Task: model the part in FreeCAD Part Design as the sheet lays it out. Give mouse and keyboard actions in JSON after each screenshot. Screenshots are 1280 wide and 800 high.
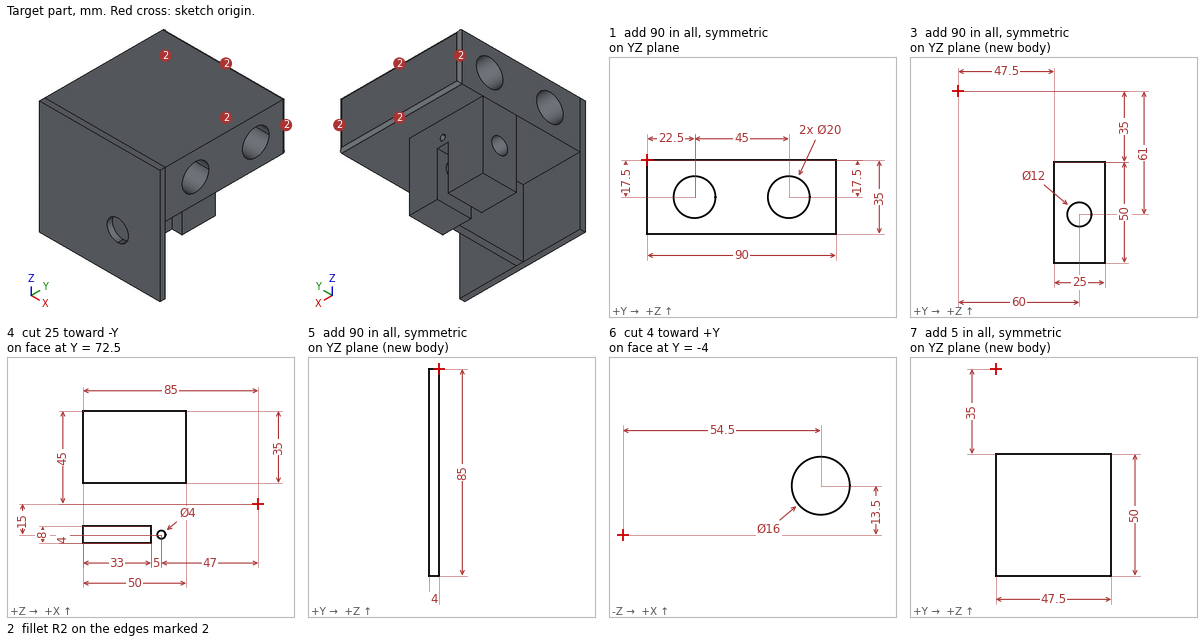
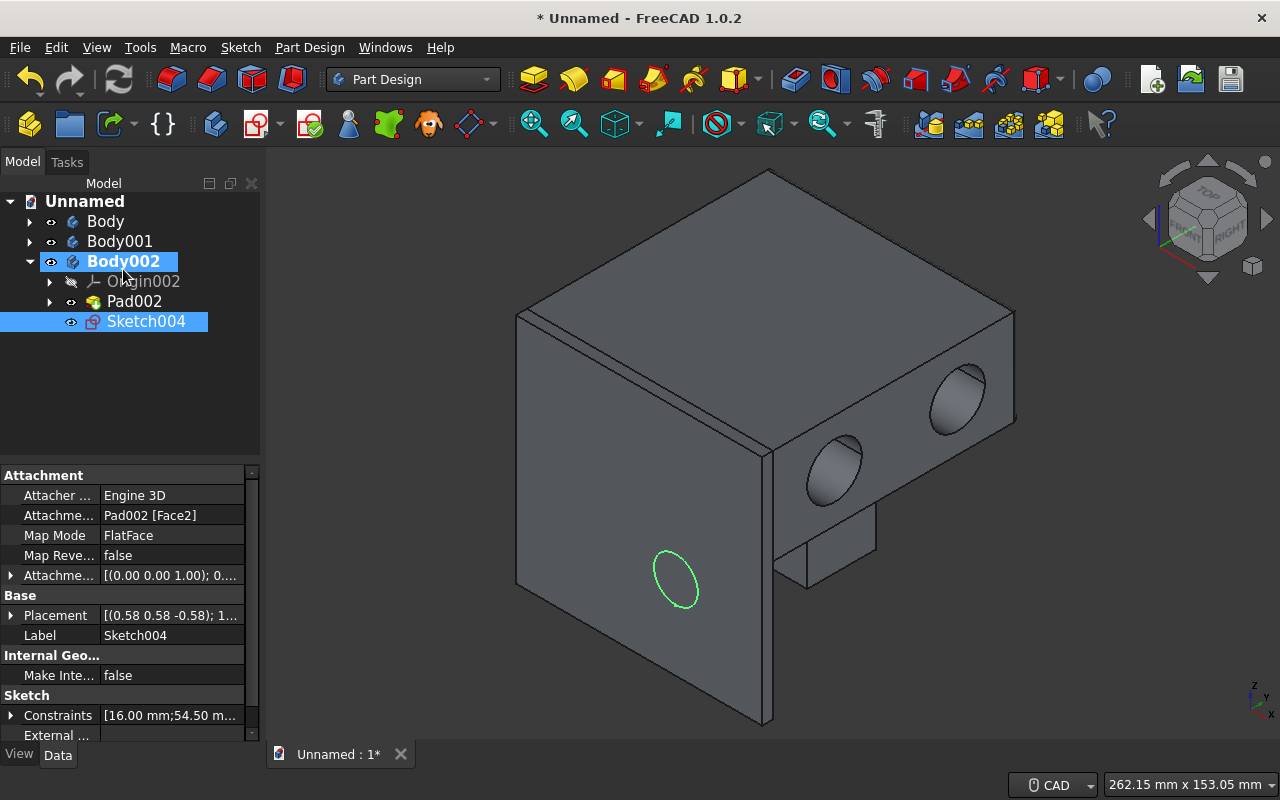
{"action": "left_click", "coordinate": [796, 80]}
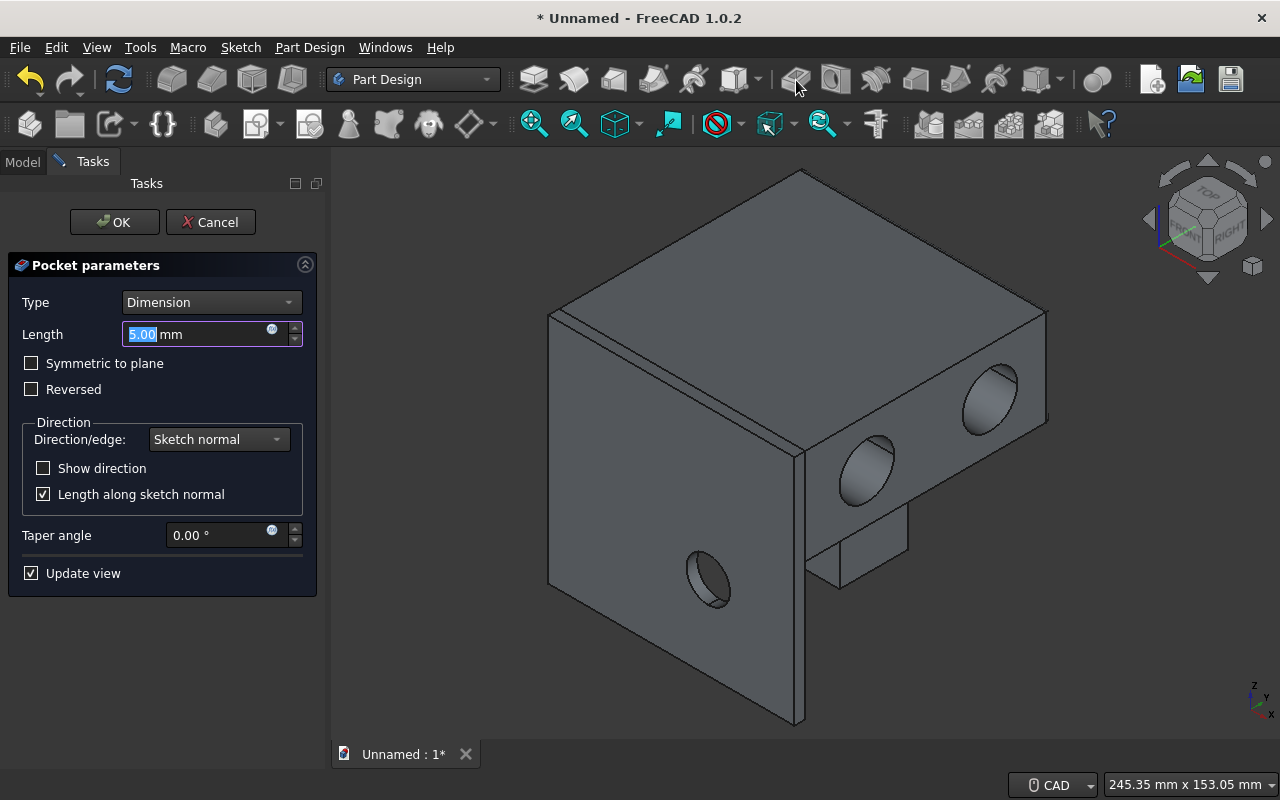
{"action": "type", "text": "4"}
{"action": "key", "text": "Tab"}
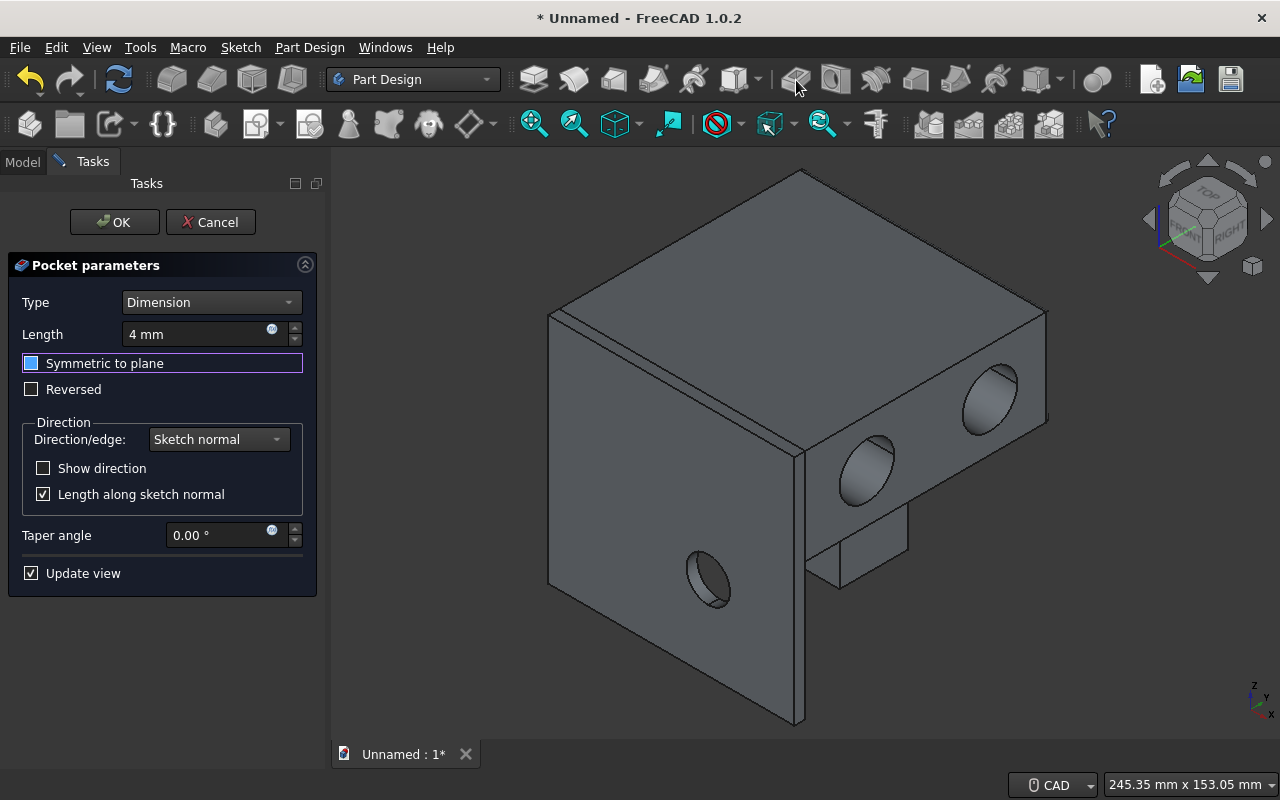
{"action": "left_click", "coordinate": [115, 222]}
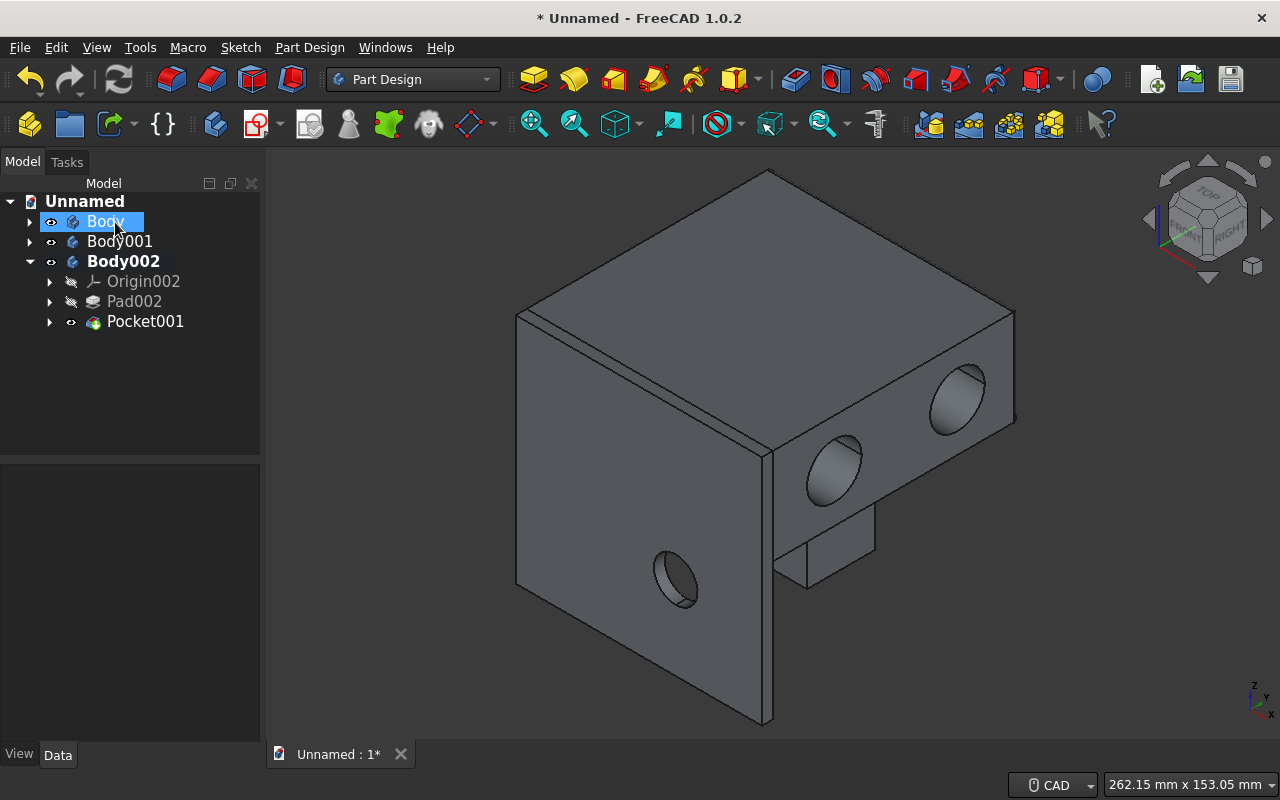
{"action": "left_click", "coordinate": [216, 124]}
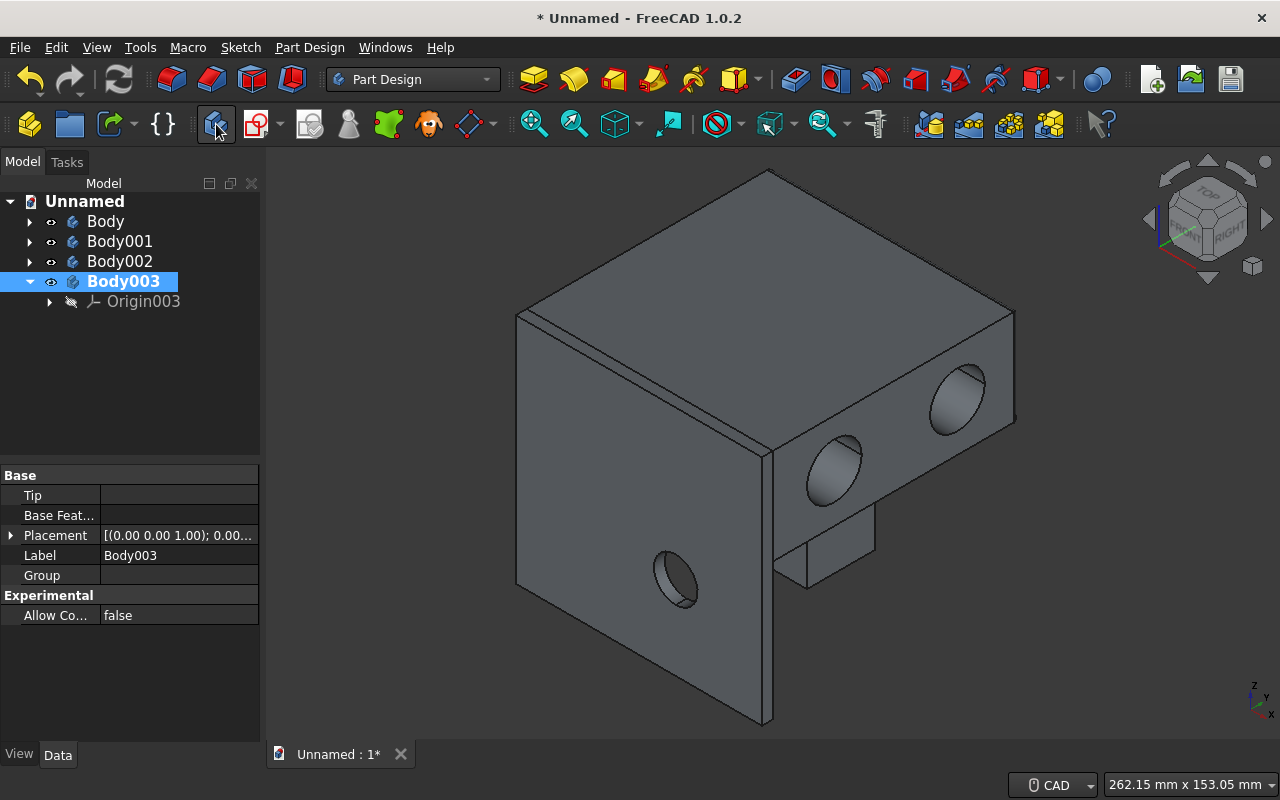
{"action": "left_click", "coordinate": [306, 699]}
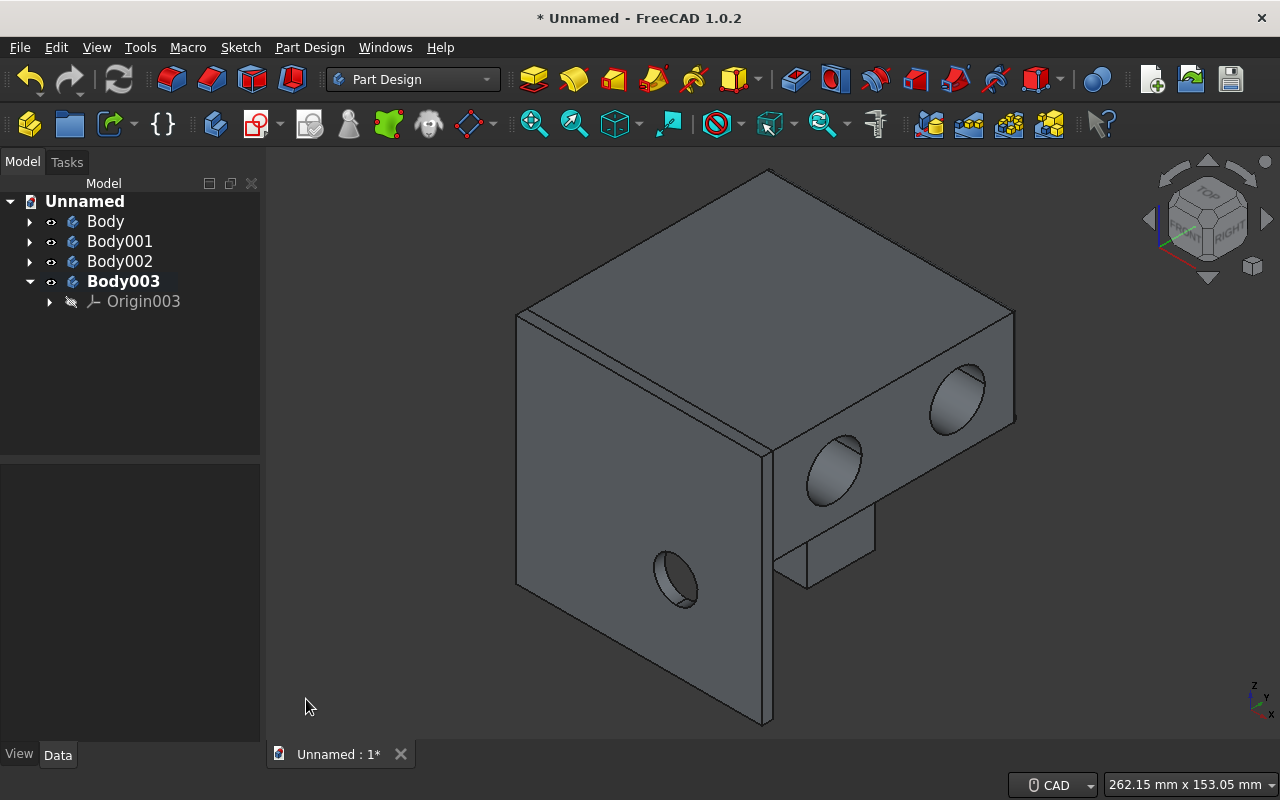
{"action": "left_click", "coordinate": [256, 124]}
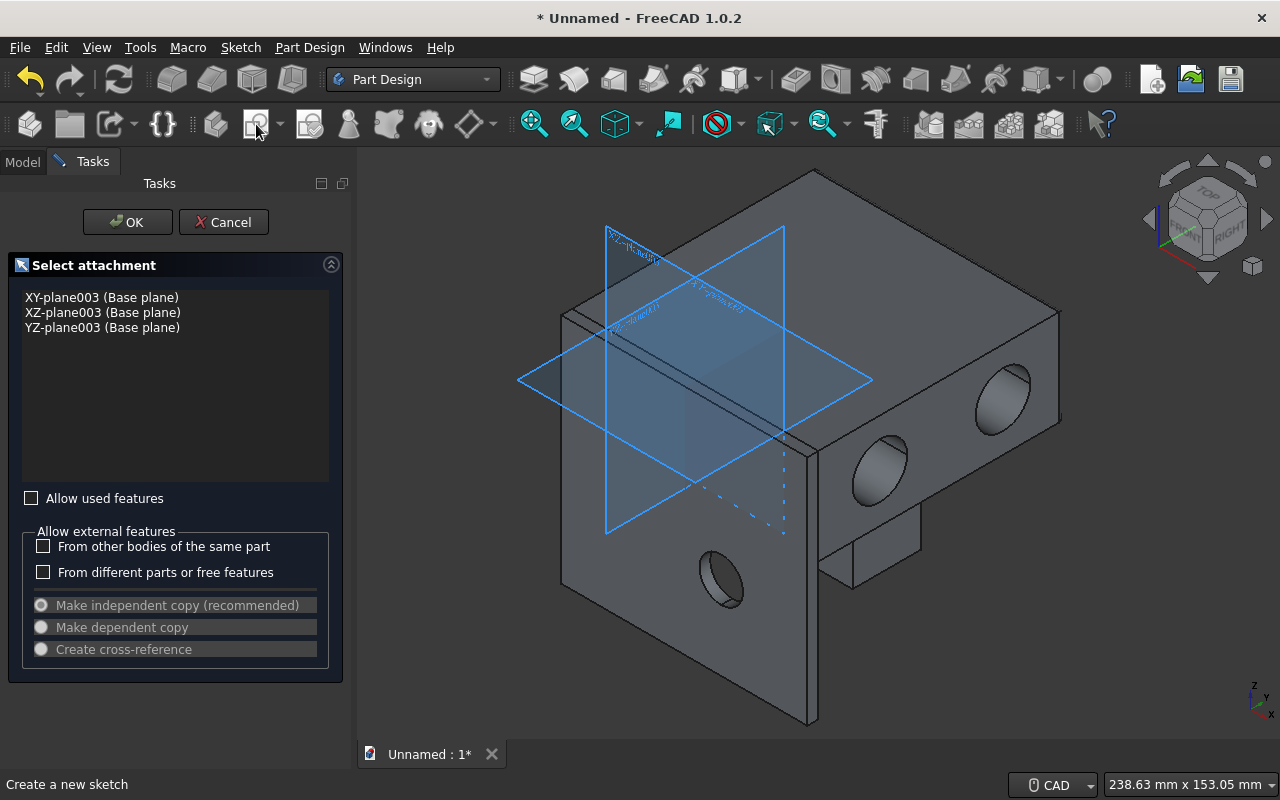
{"action": "left_click", "coordinate": [82, 328]}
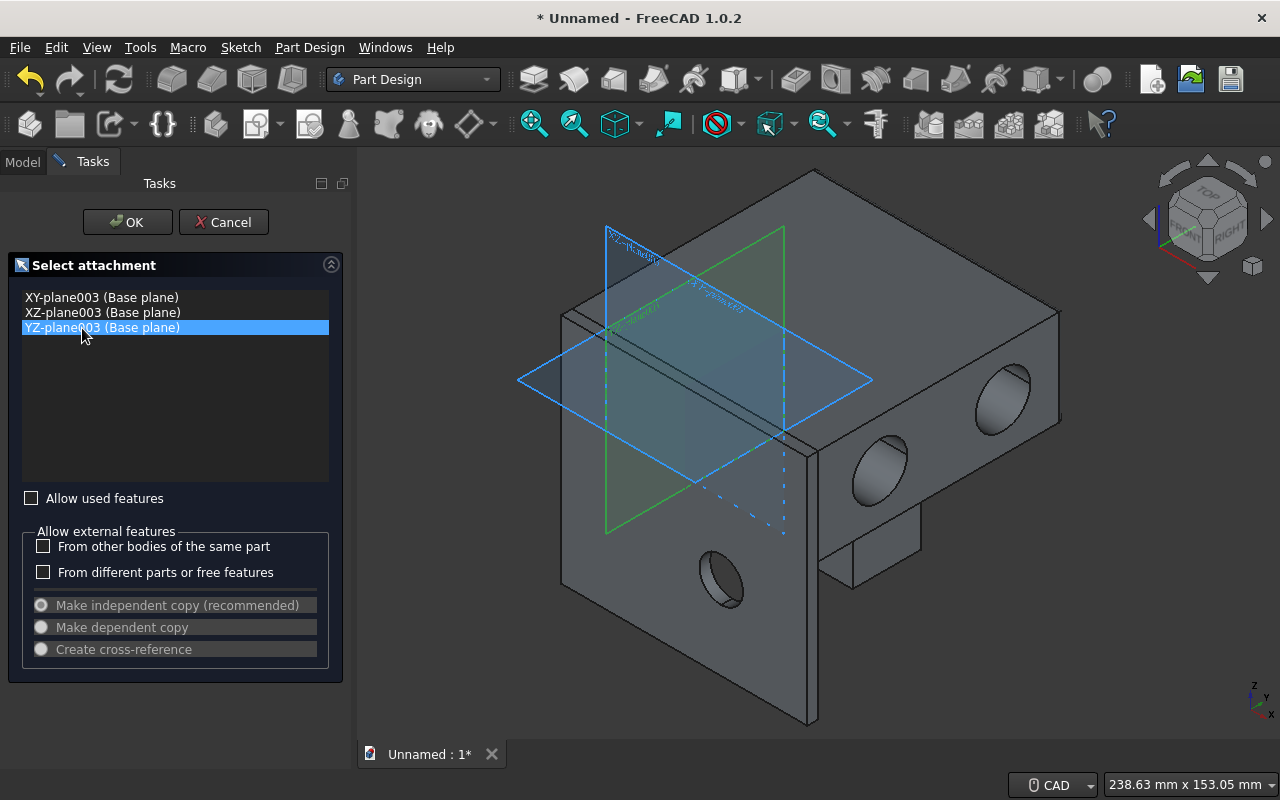
{"action": "left_click", "coordinate": [128, 222]}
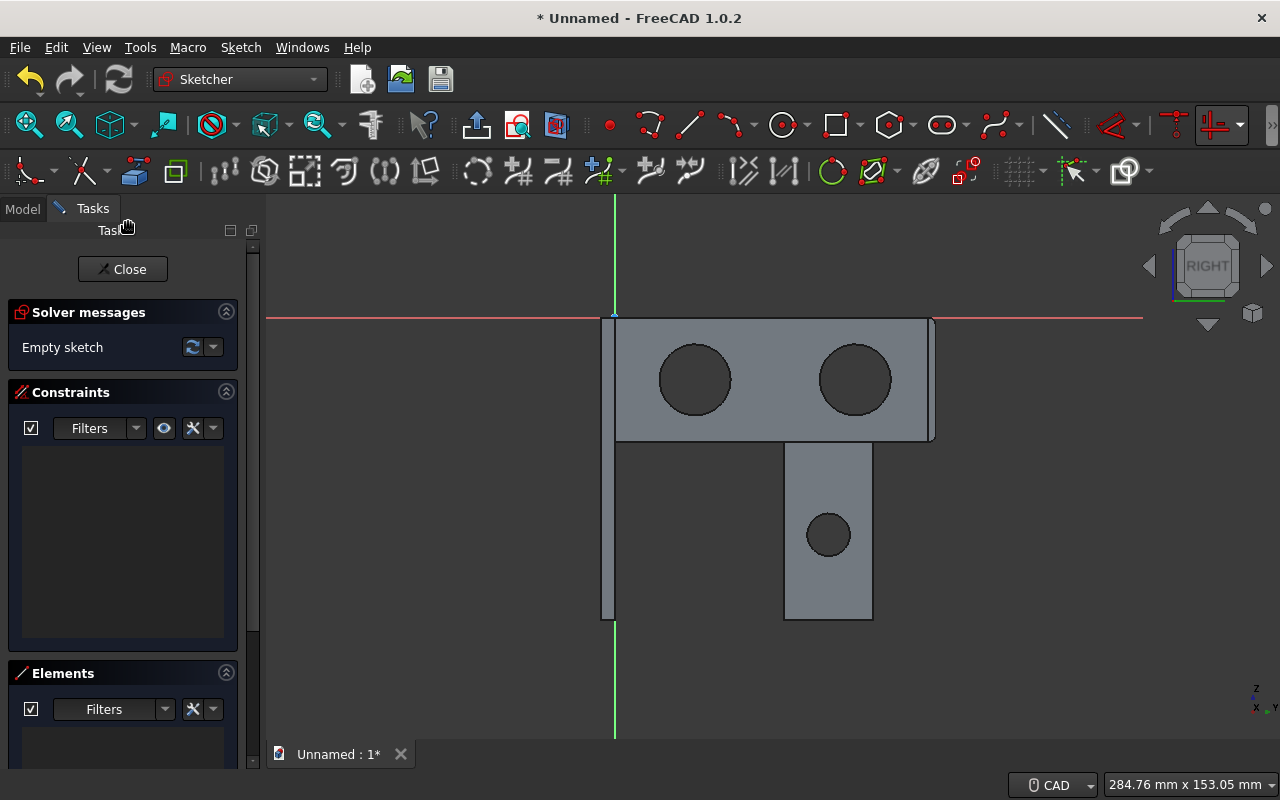
{"action": "left_click", "coordinate": [836, 126]}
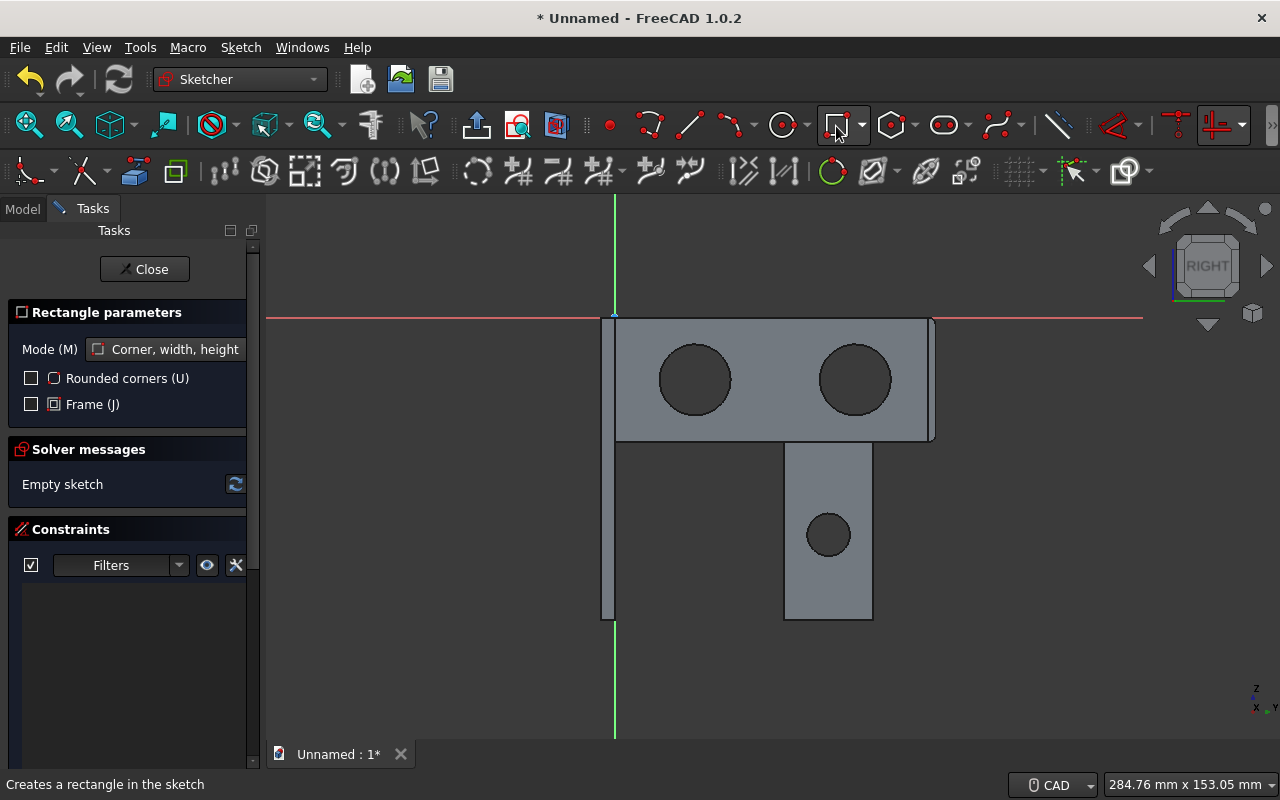
{"action": "left_click", "coordinate": [615, 442]}
{"action": "mouse_move", "coordinate": [784, 620]}